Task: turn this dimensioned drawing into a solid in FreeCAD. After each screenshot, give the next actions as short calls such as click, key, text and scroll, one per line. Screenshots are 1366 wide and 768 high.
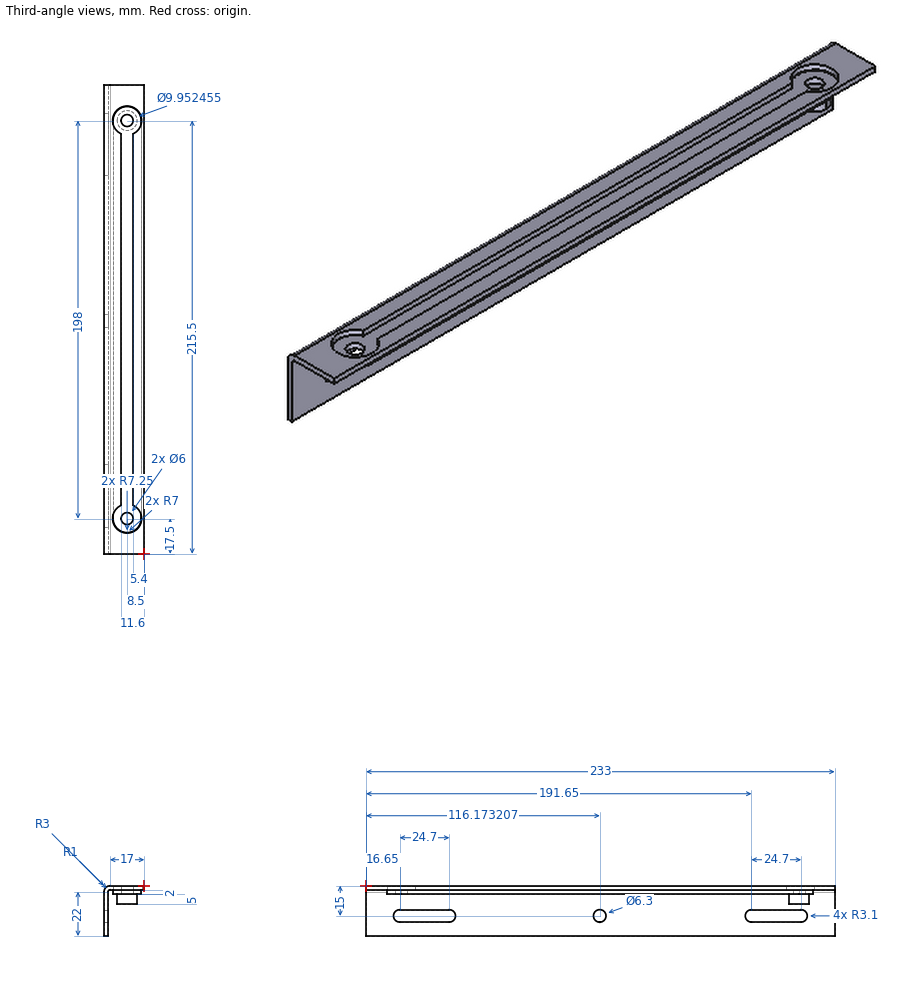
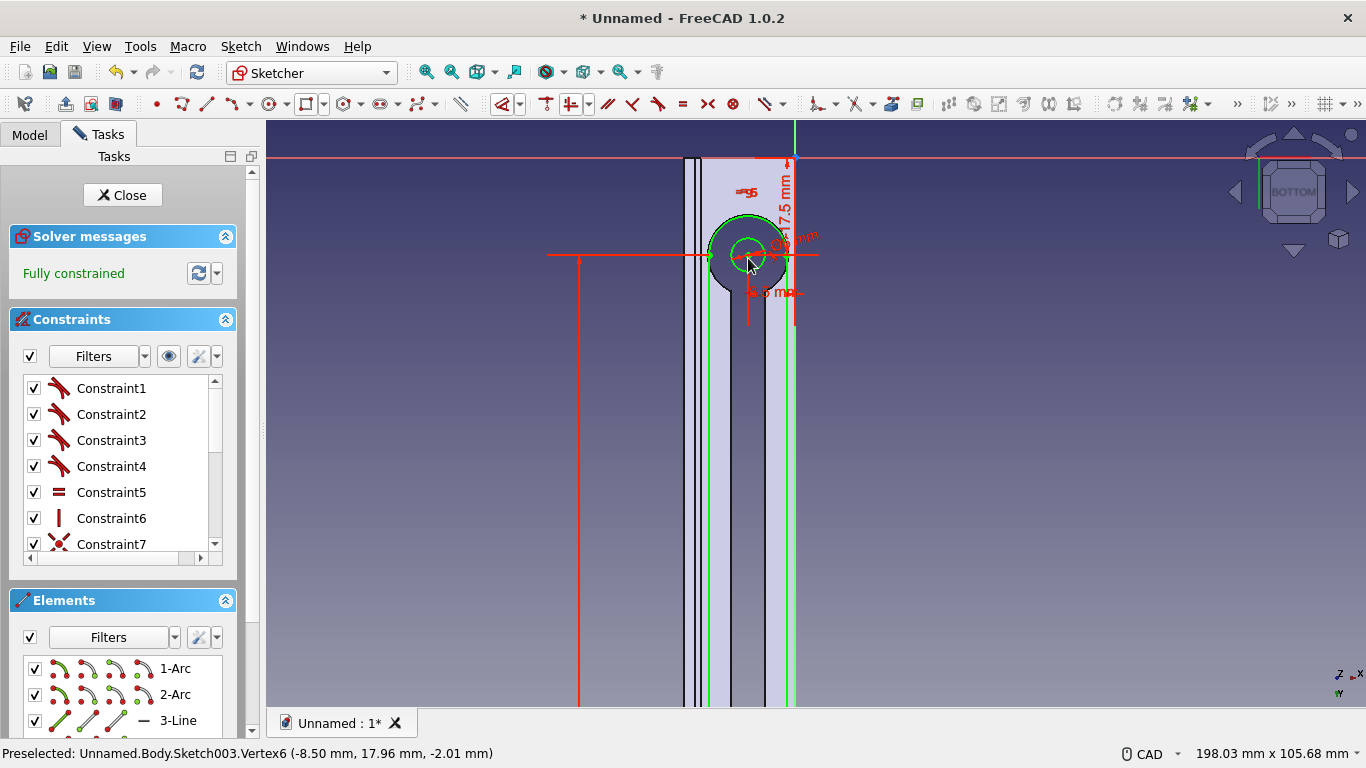
click(123, 195)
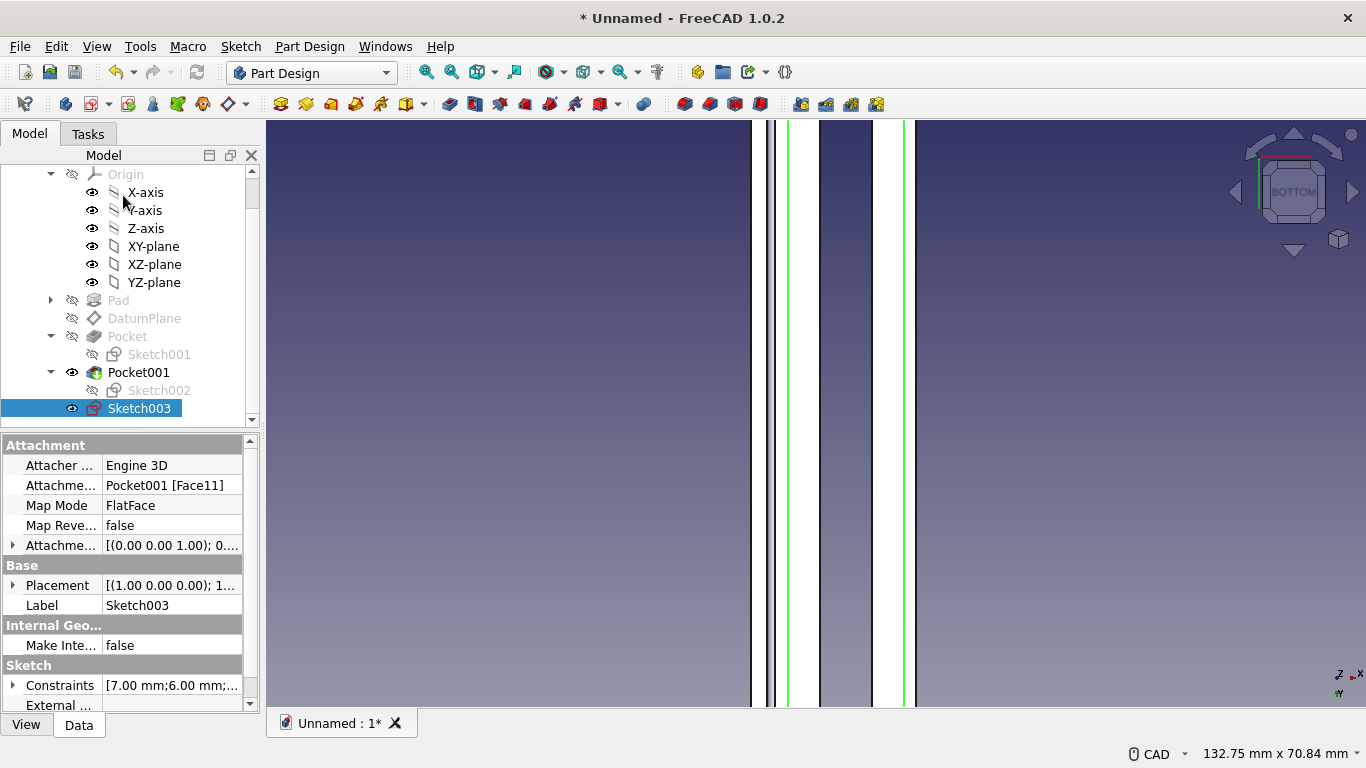
click(281, 104)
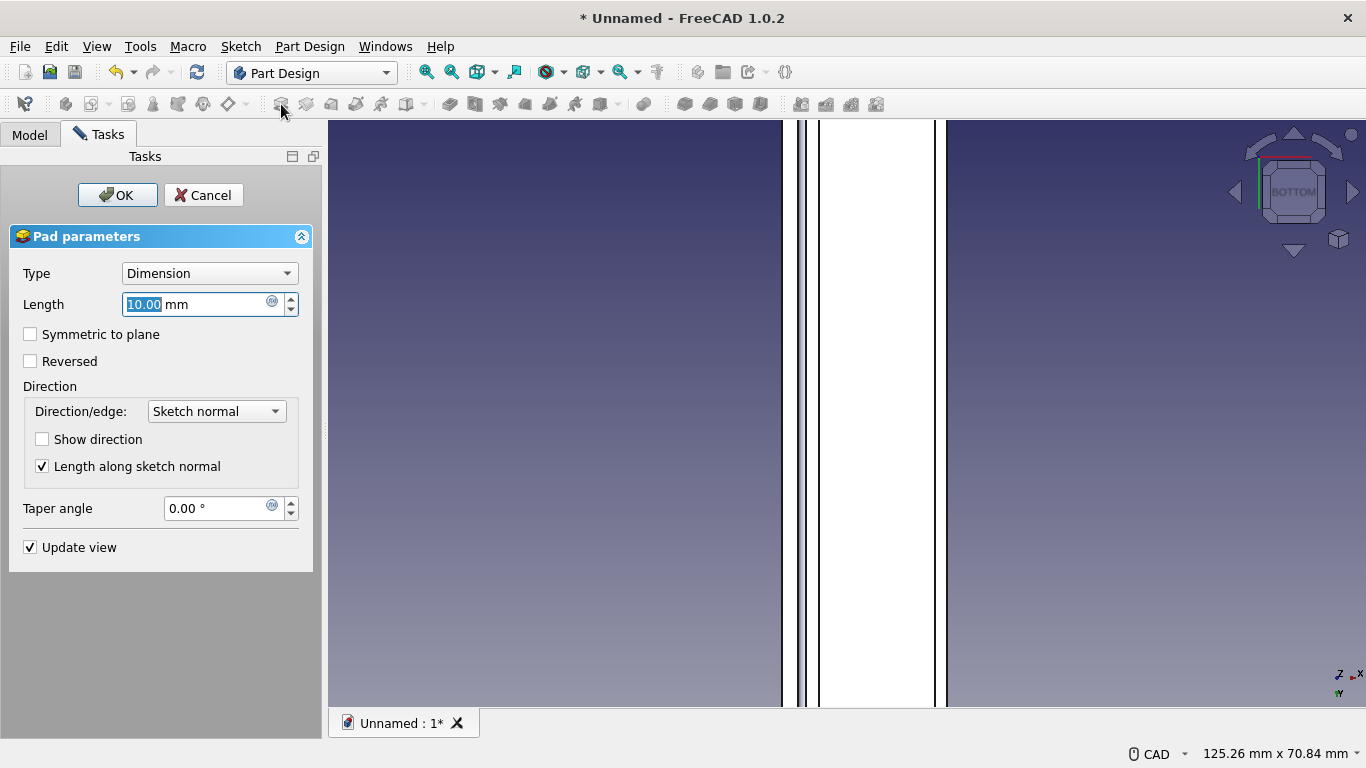
text(2)
key(Tab)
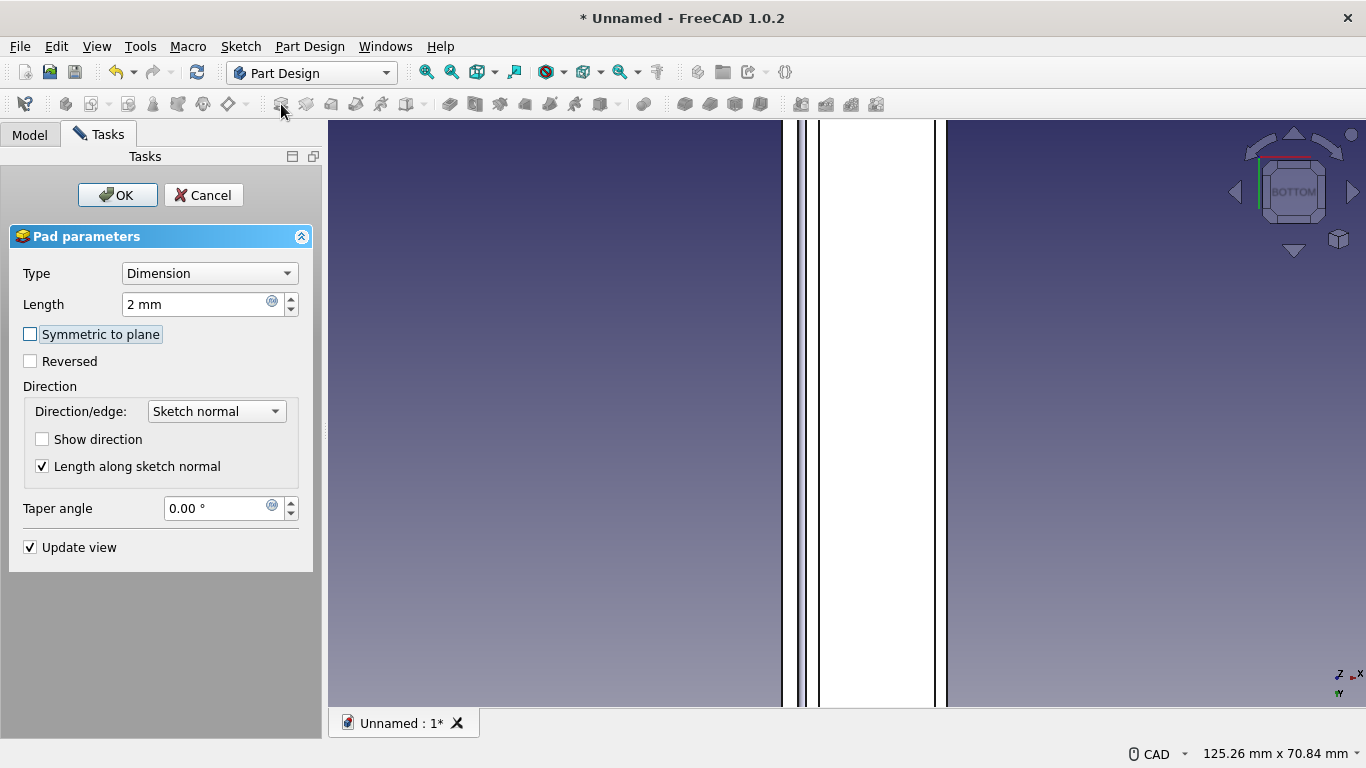
click(118, 195)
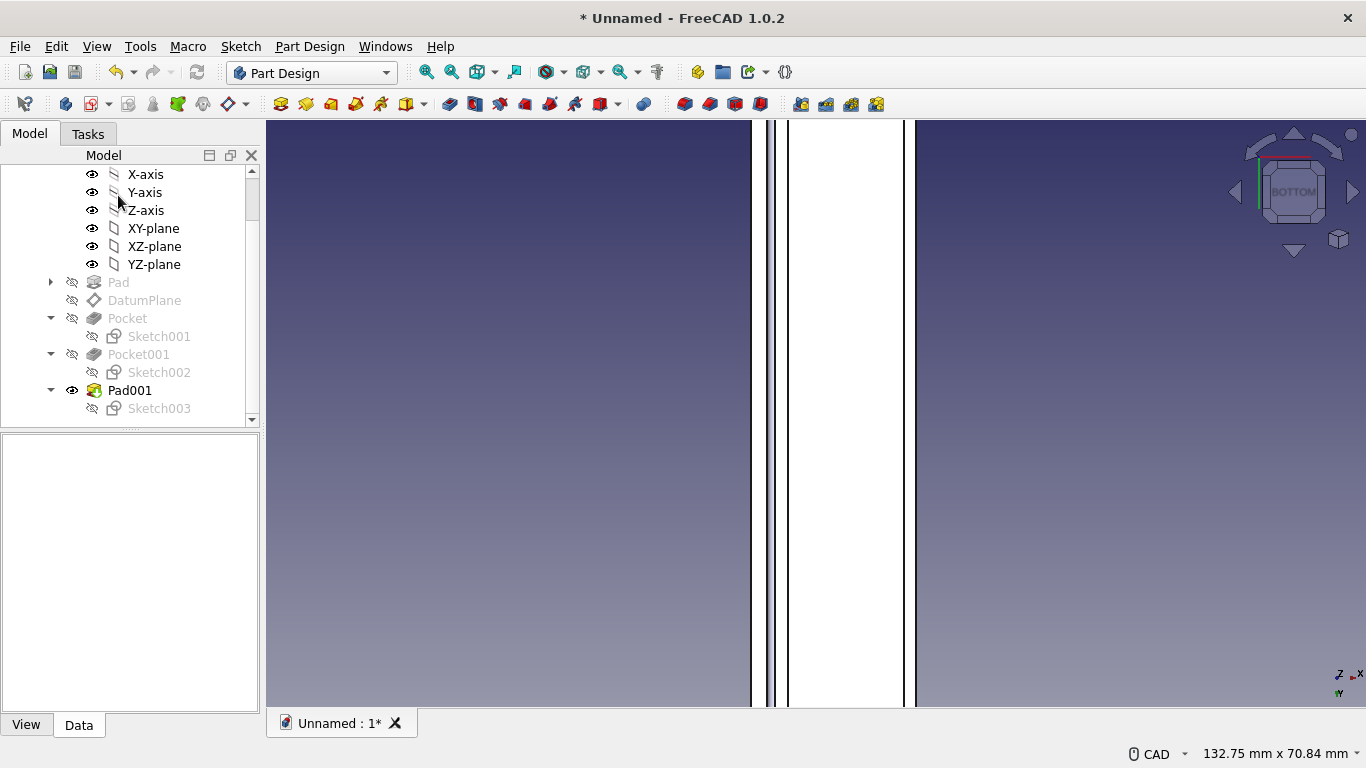
click(427, 72)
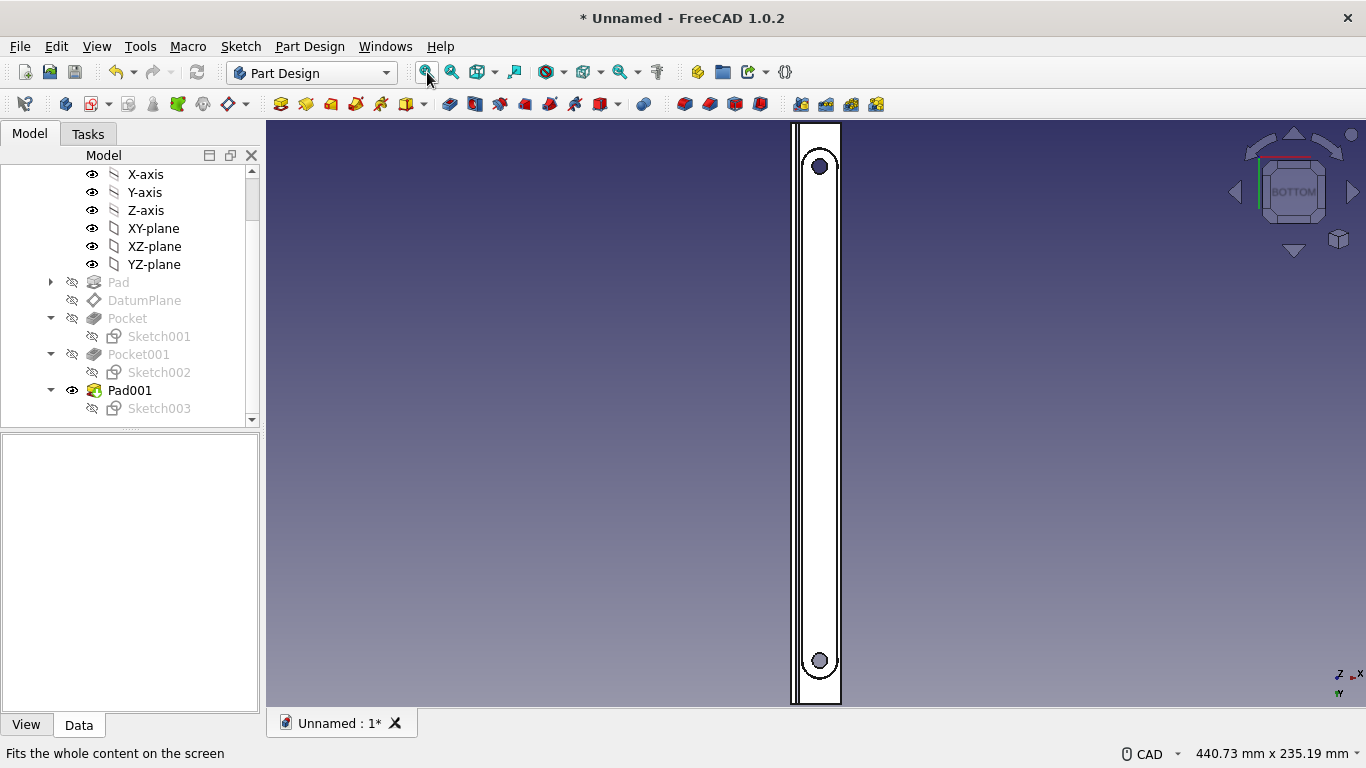
click(66, 104)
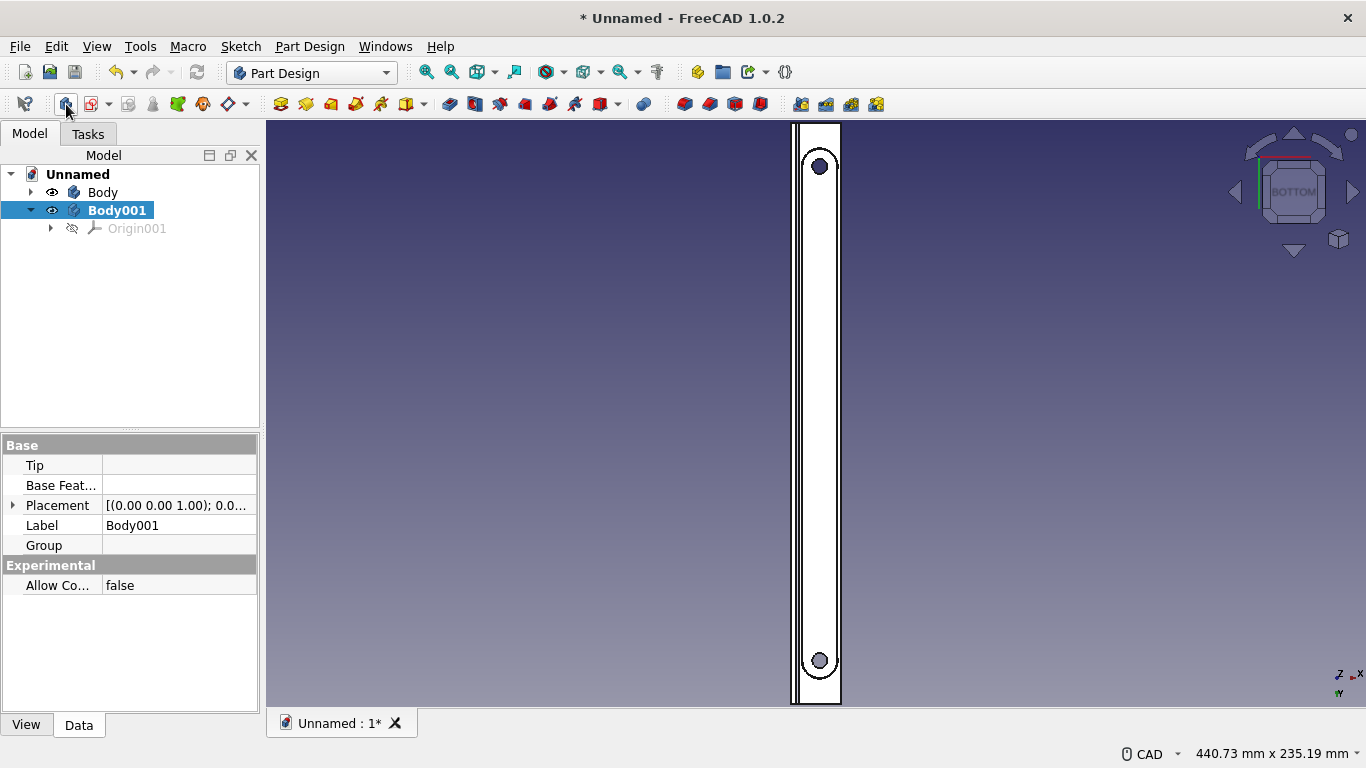
click(51, 228)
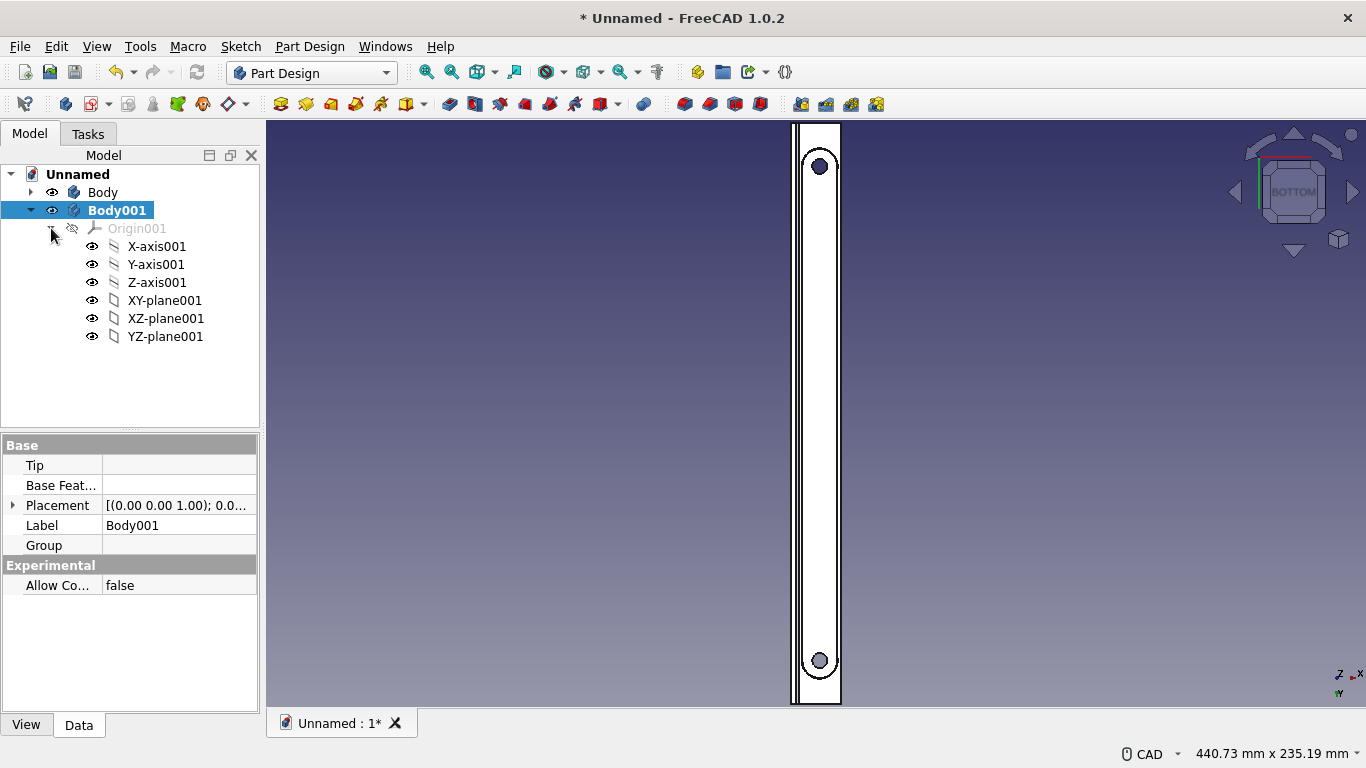
click(137, 300)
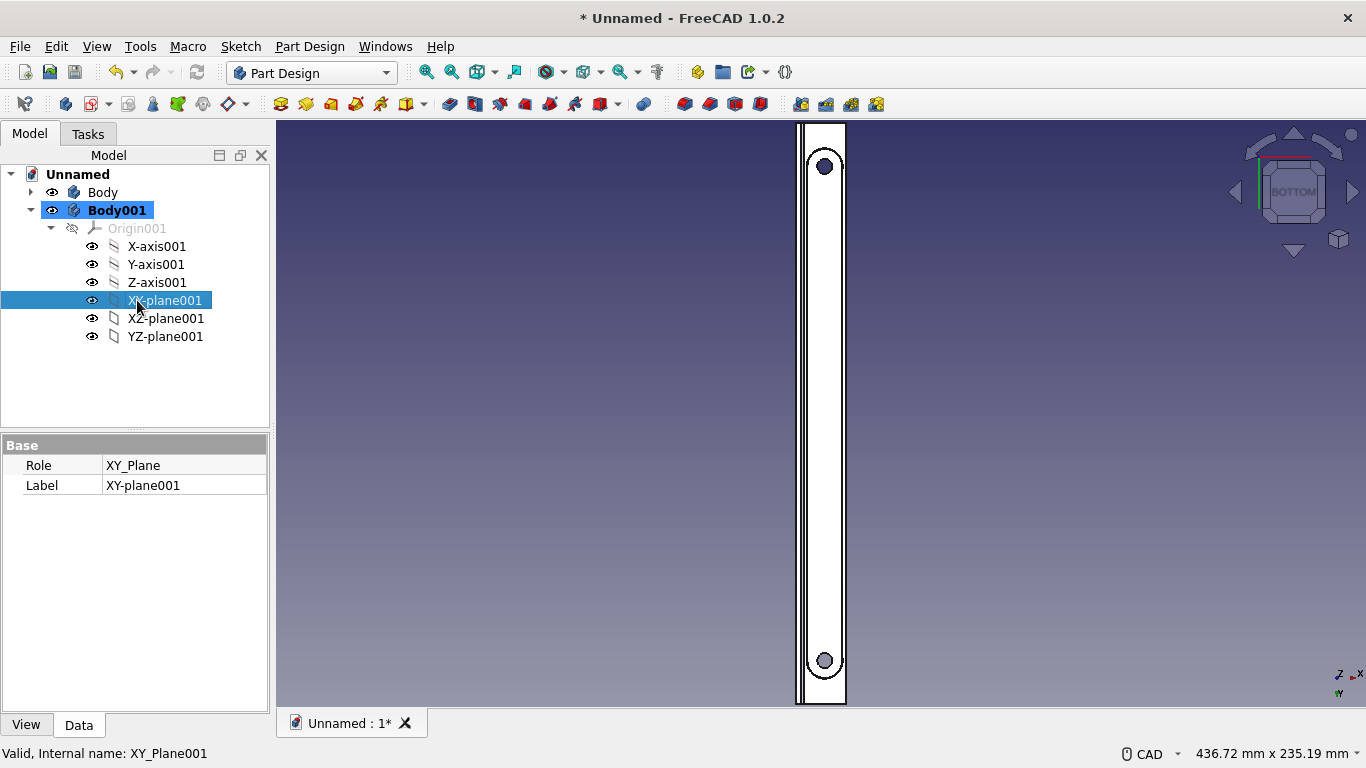
click(228, 104)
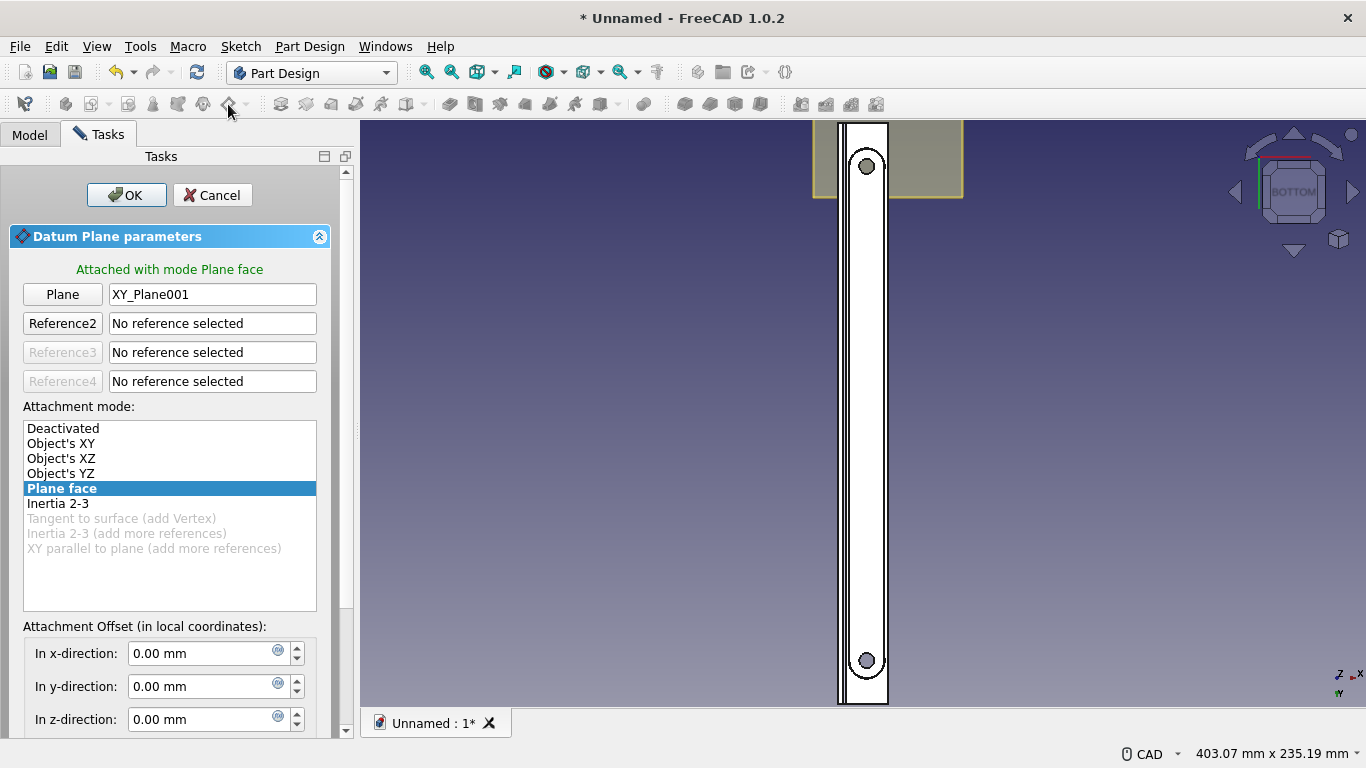
triple_click(210, 720)